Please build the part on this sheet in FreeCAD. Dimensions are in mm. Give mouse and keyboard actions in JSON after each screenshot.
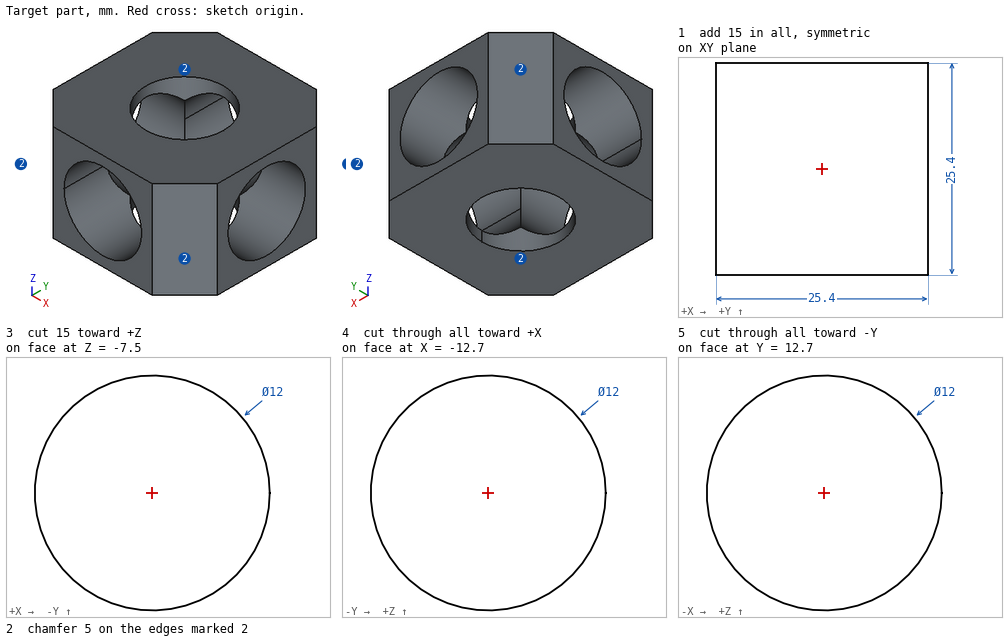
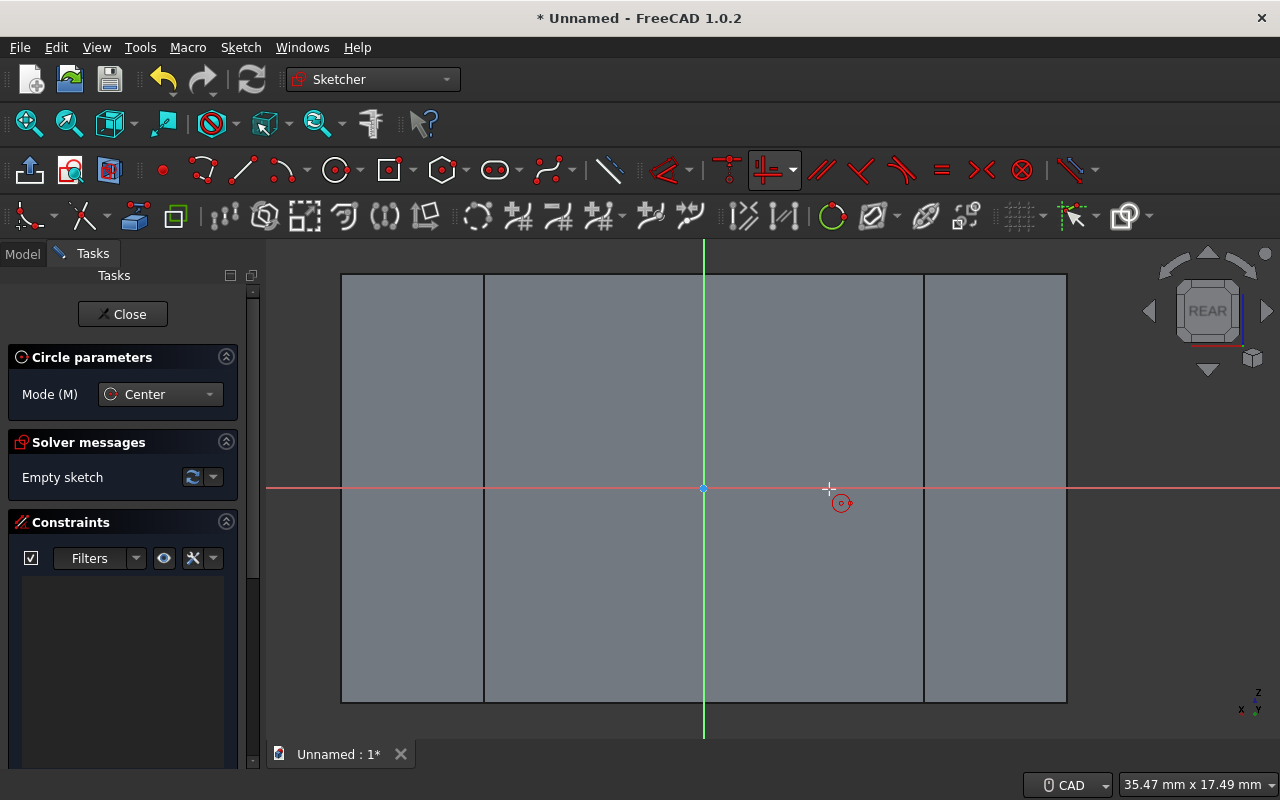
{"action": "left_click", "coordinate": [704, 488]}
{"action": "left_click", "coordinate": [825, 367]}
{"action": "key", "text": "Escape"}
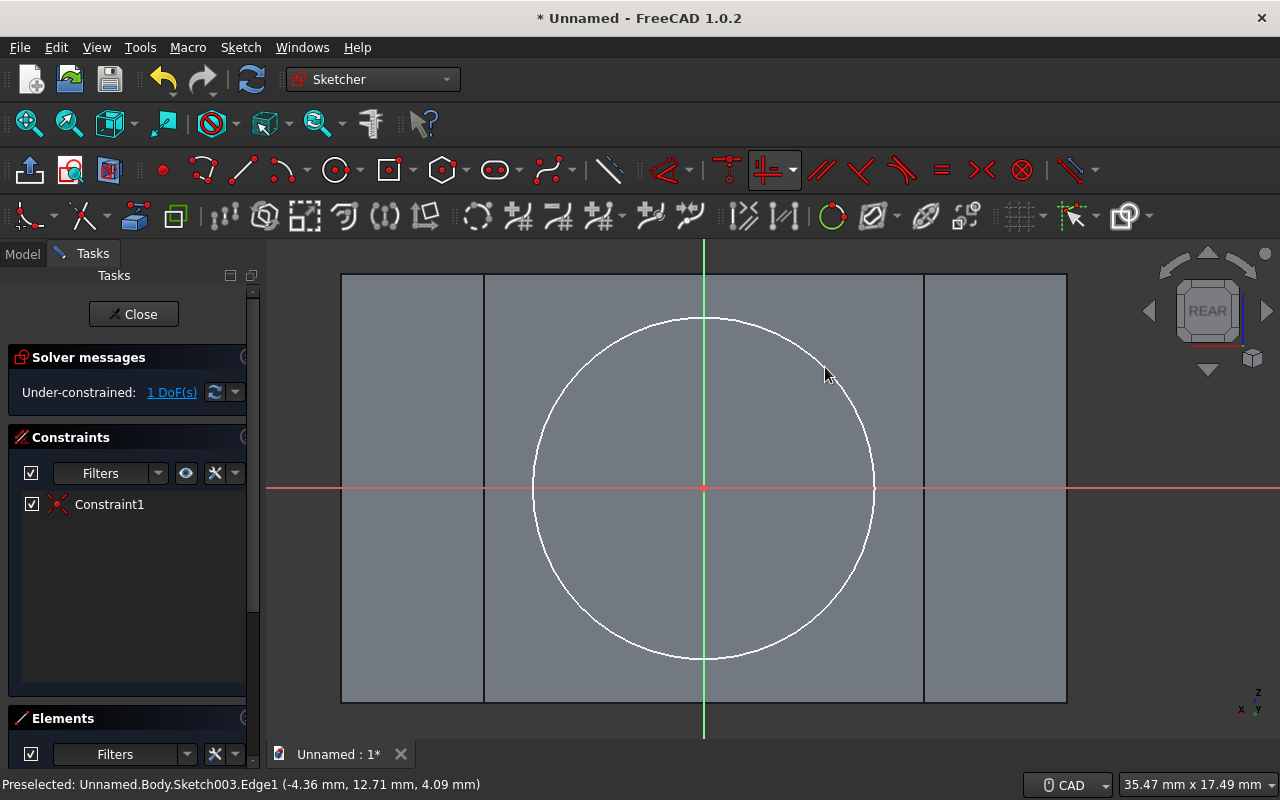
{"action": "key", "text": "d"}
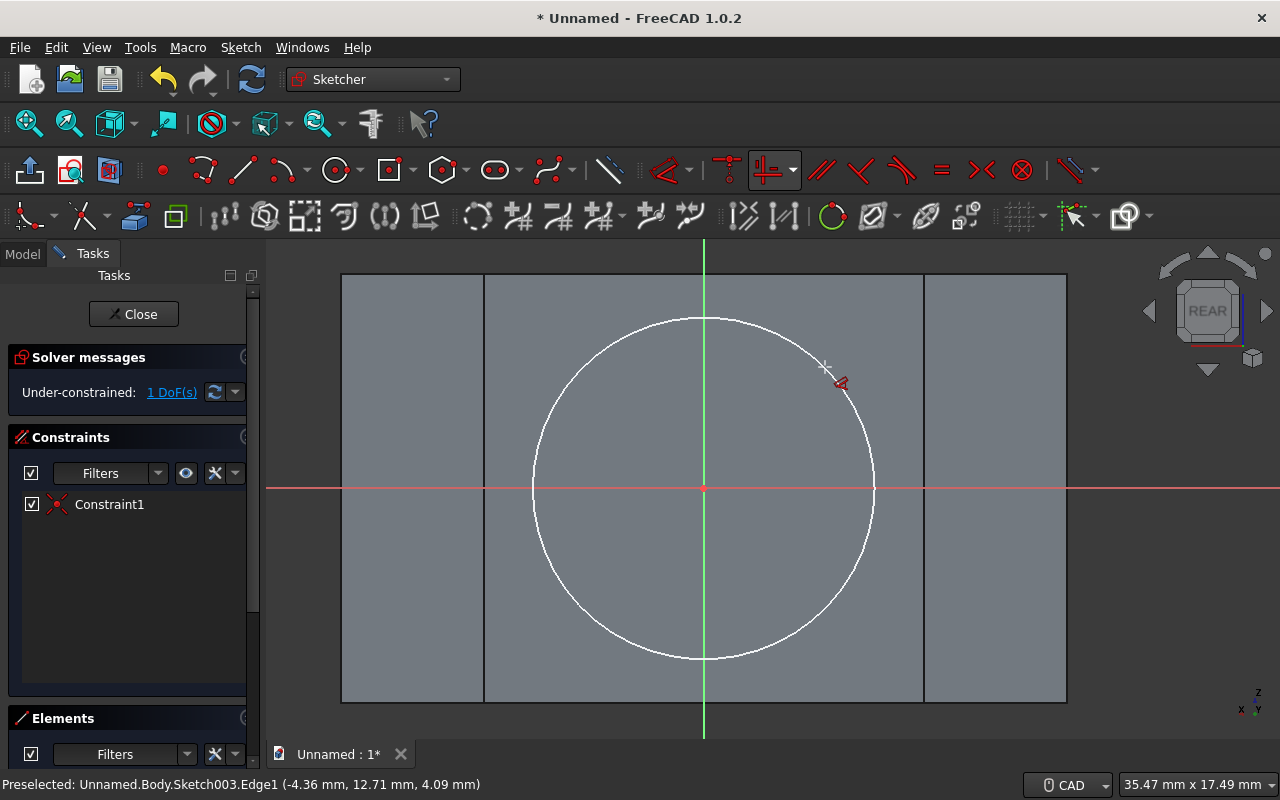
{"action": "left_click", "coordinate": [824, 367]}
{"action": "left_click", "coordinate": [847, 344]}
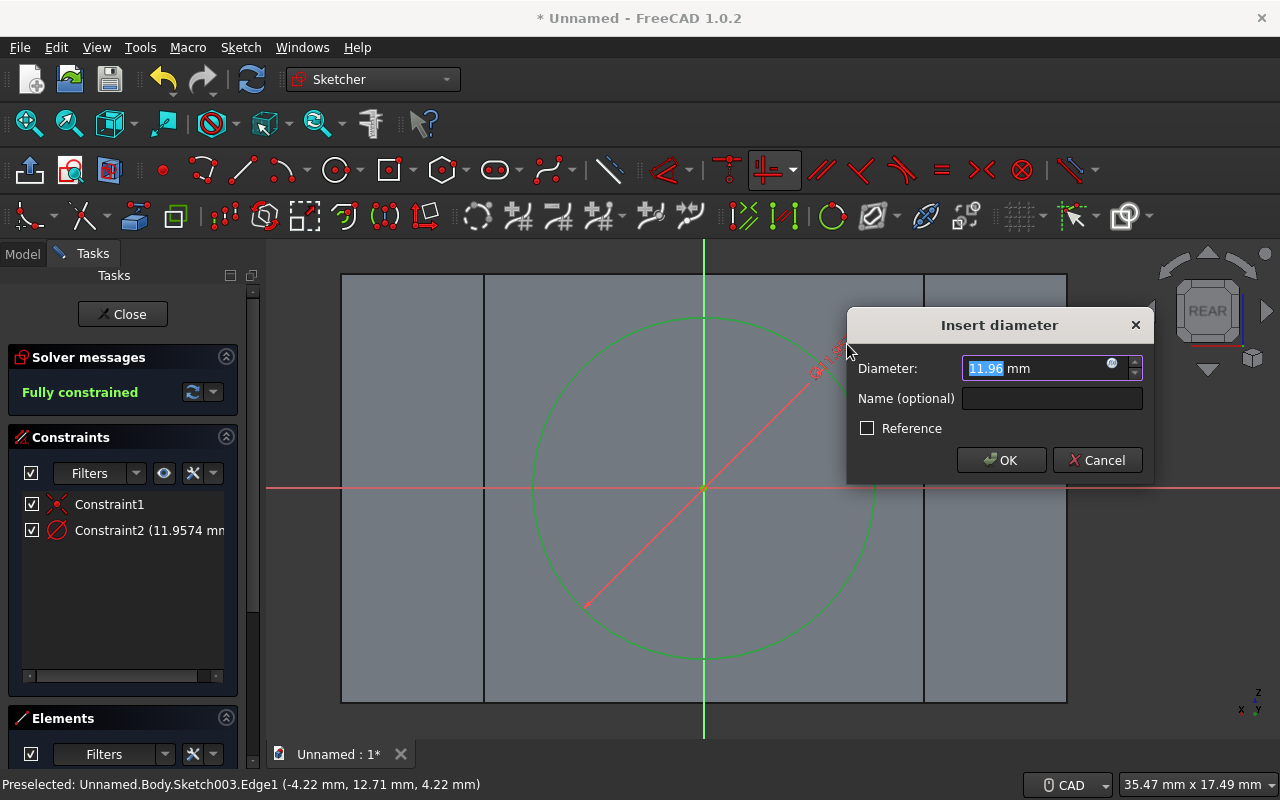
{"action": "type", "text": "12"}
{"action": "key", "text": "Return"}
{"action": "key", "text": "Escape"}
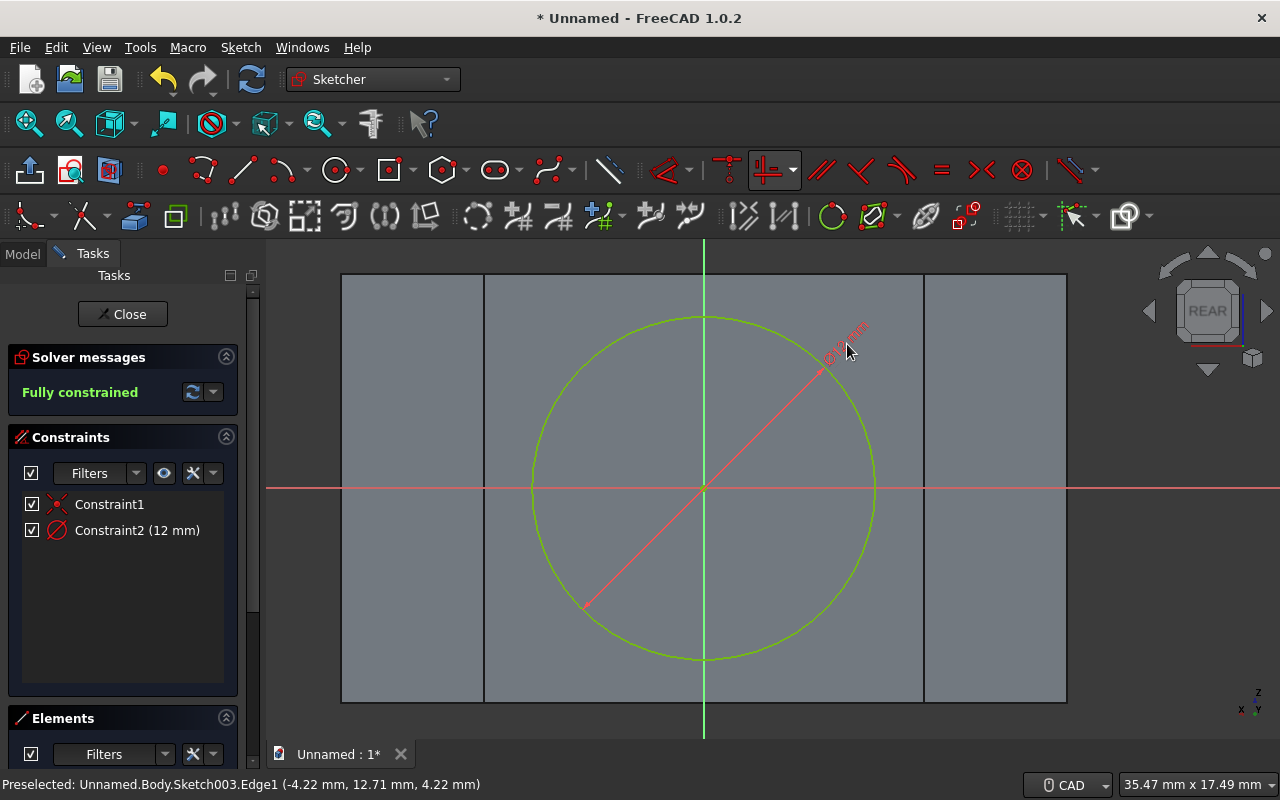
{"action": "left_click", "coordinate": [123, 314]}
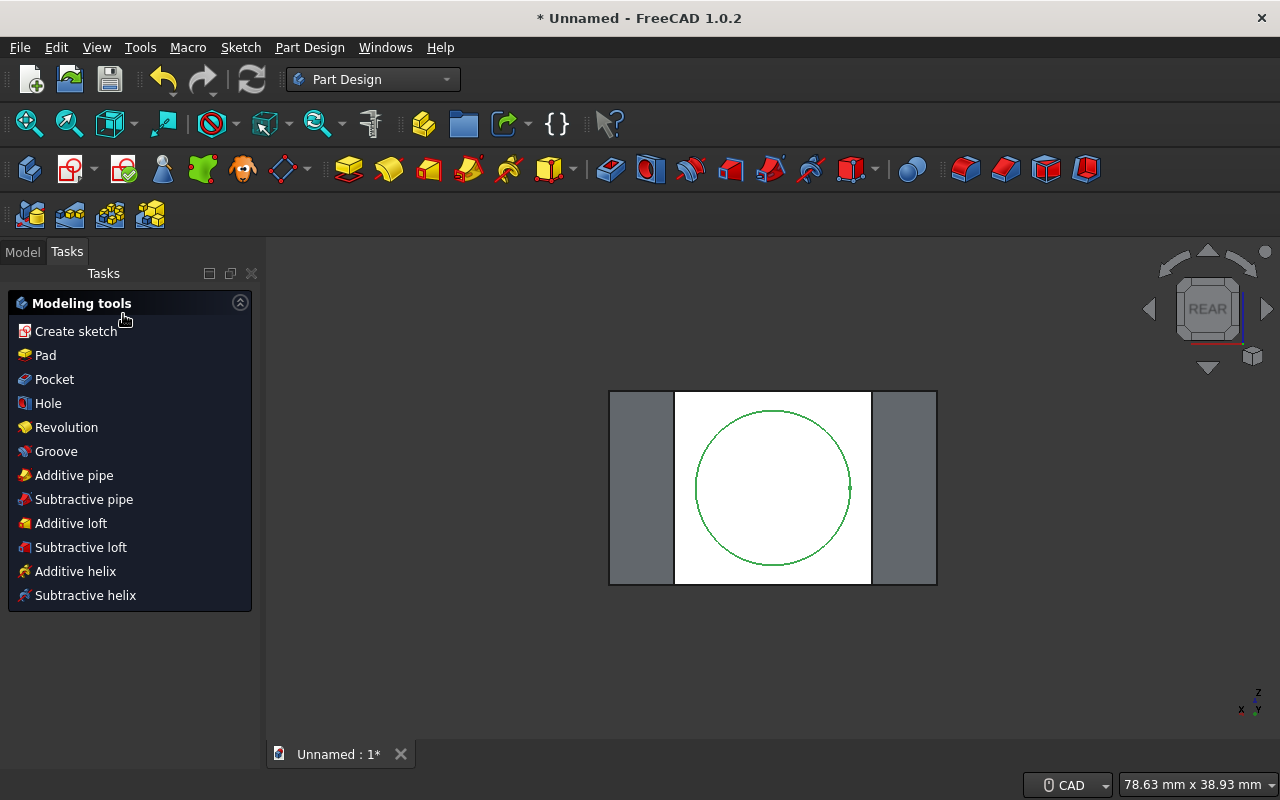
{"action": "left_click", "coordinate": [612, 170]}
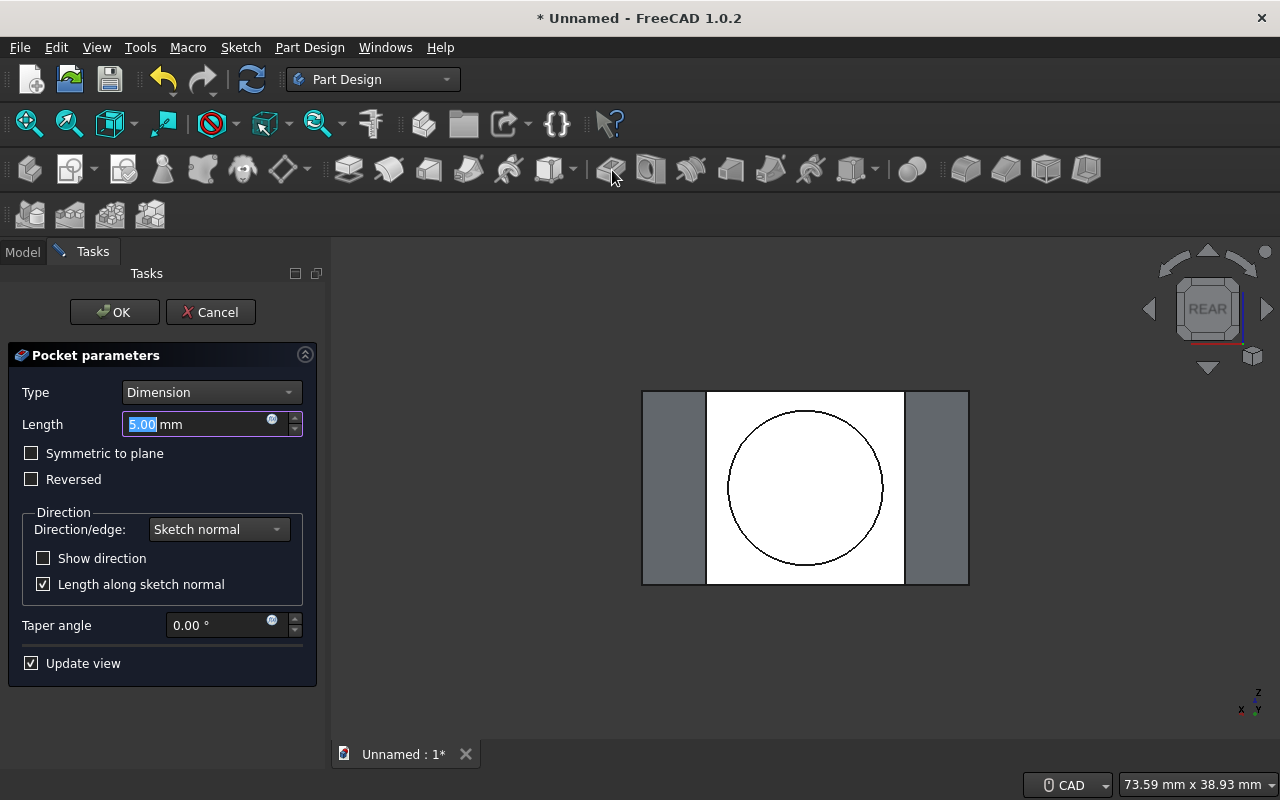
{"action": "left_click", "coordinate": [212, 392]}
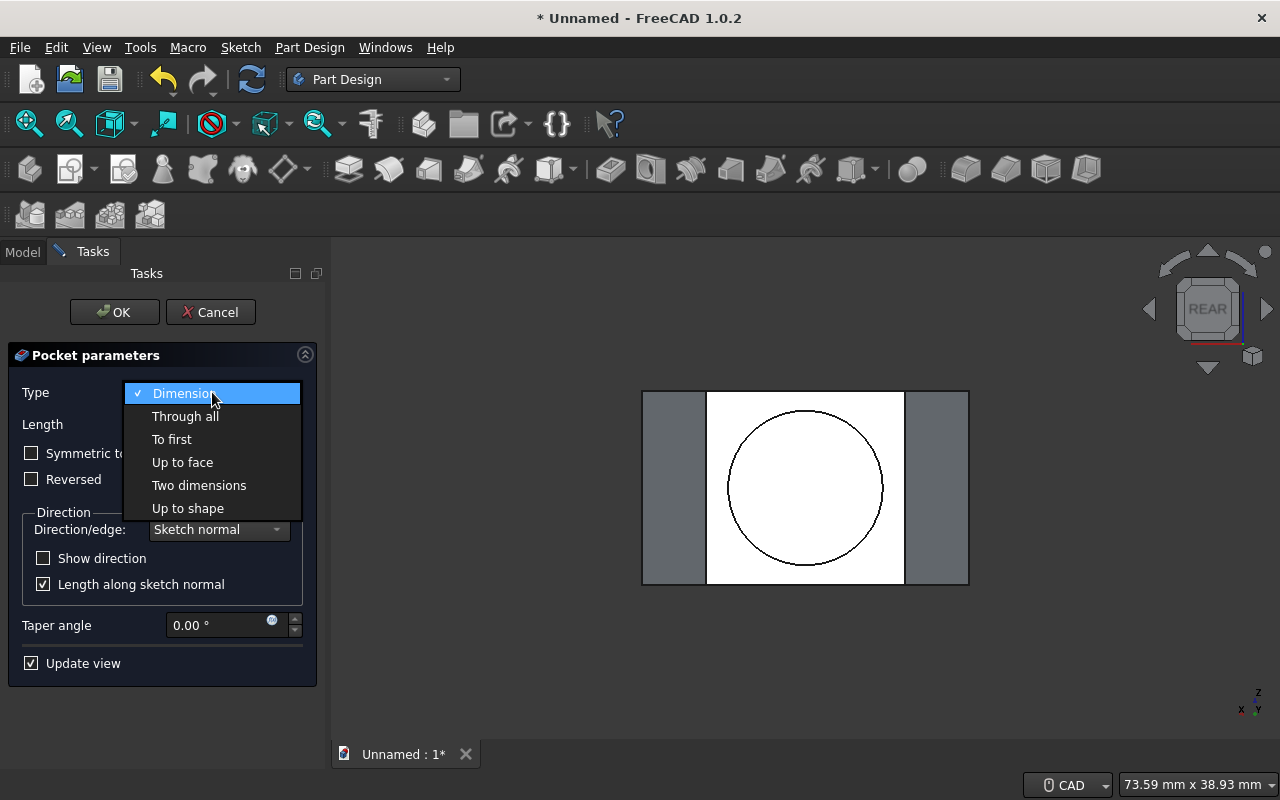
{"action": "left_click", "coordinate": [212, 416]}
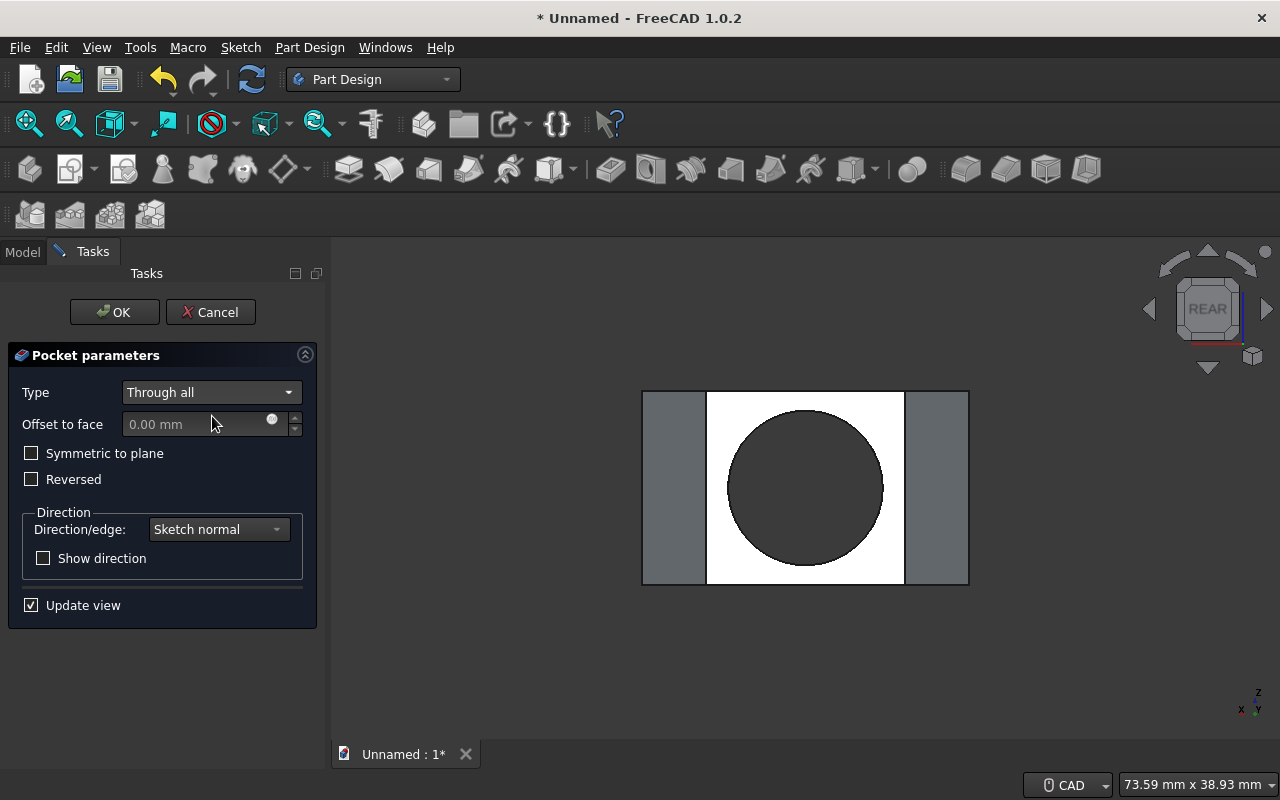
{"action": "left_click", "coordinate": [115, 312]}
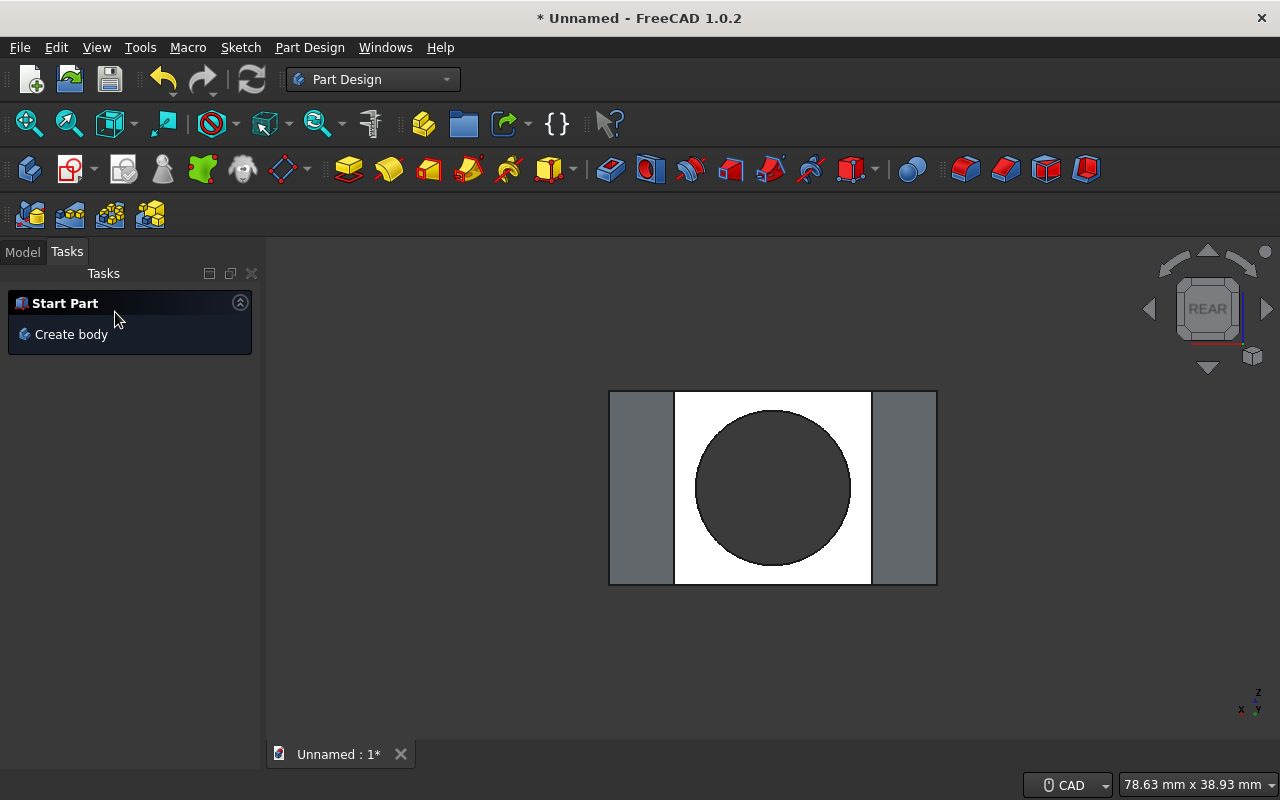
{"action": "key", "text": "0"}